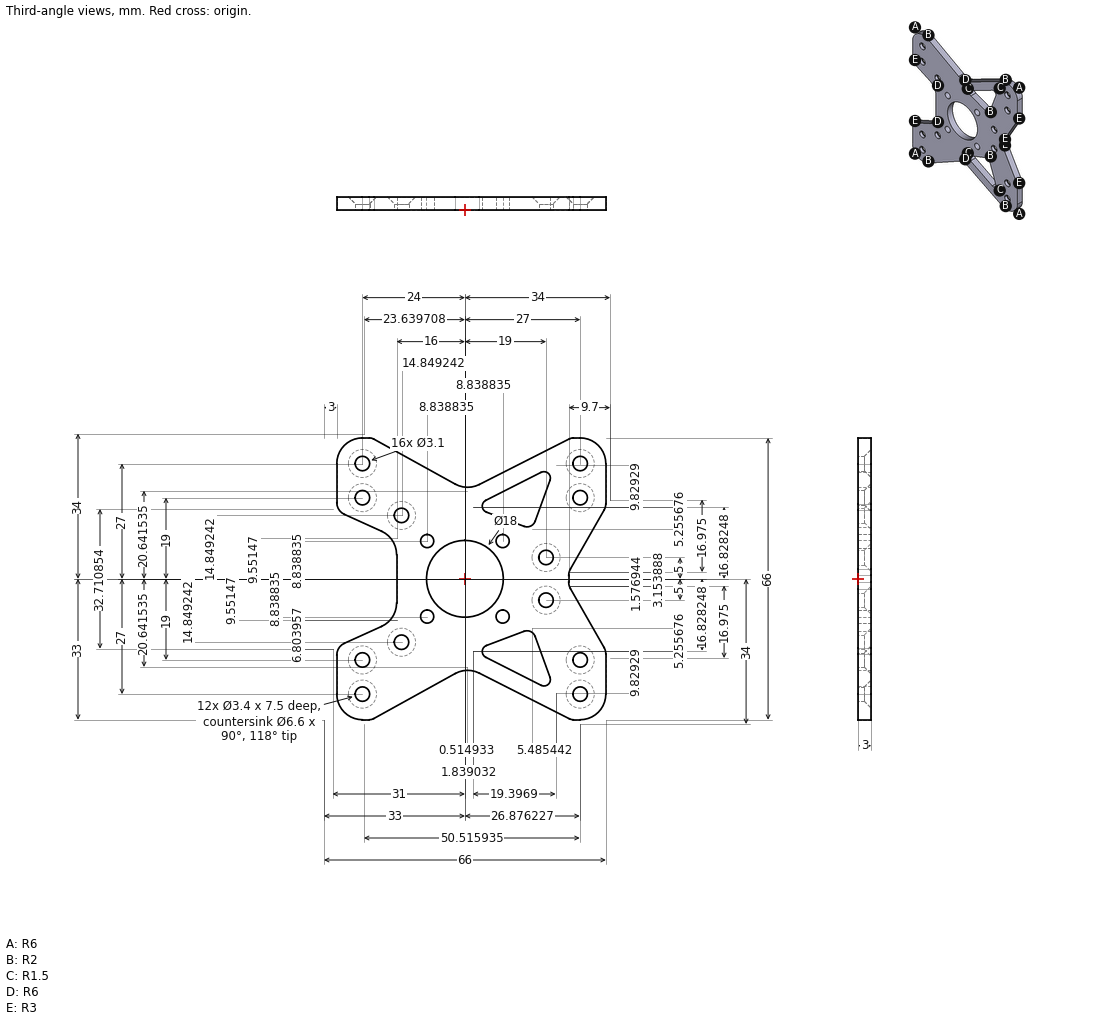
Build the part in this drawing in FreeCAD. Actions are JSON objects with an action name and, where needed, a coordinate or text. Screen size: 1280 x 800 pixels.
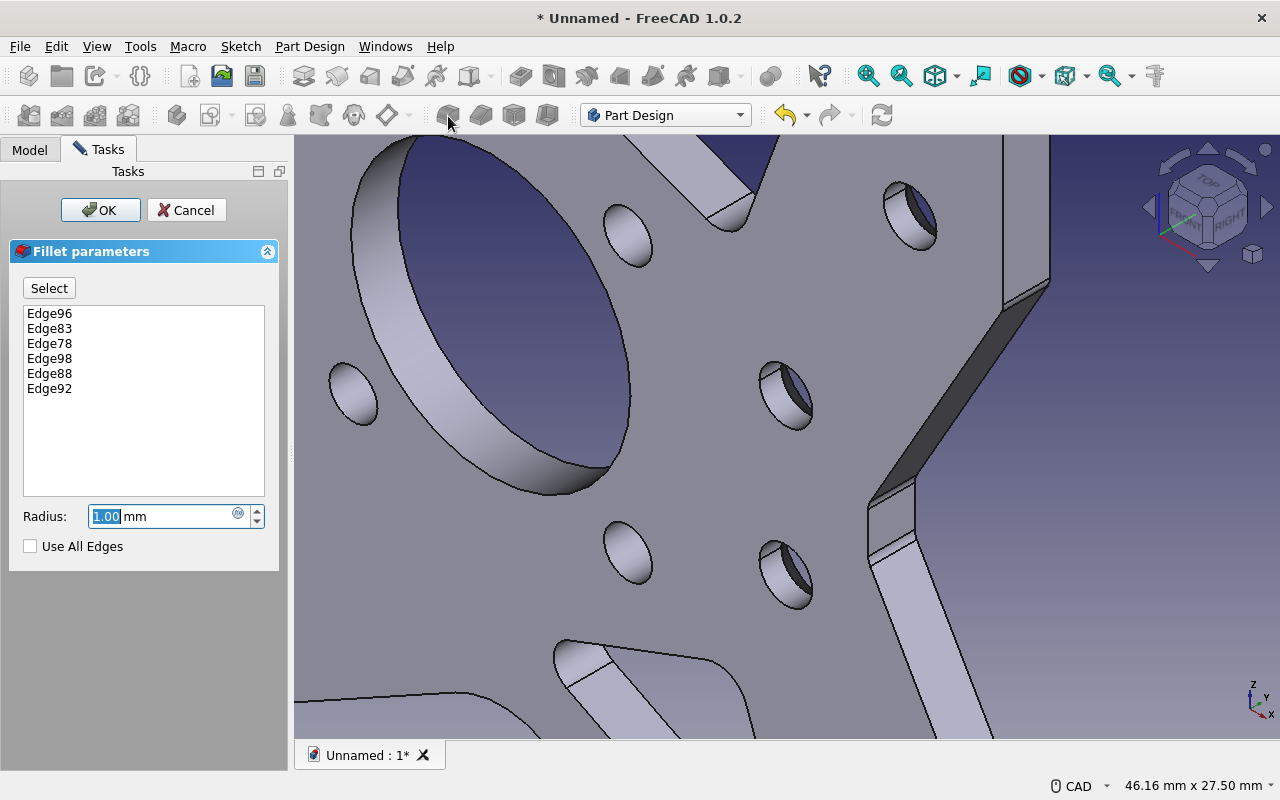
{"action": "type", "text": "3"}
{"action": "key", "text": "Tab"}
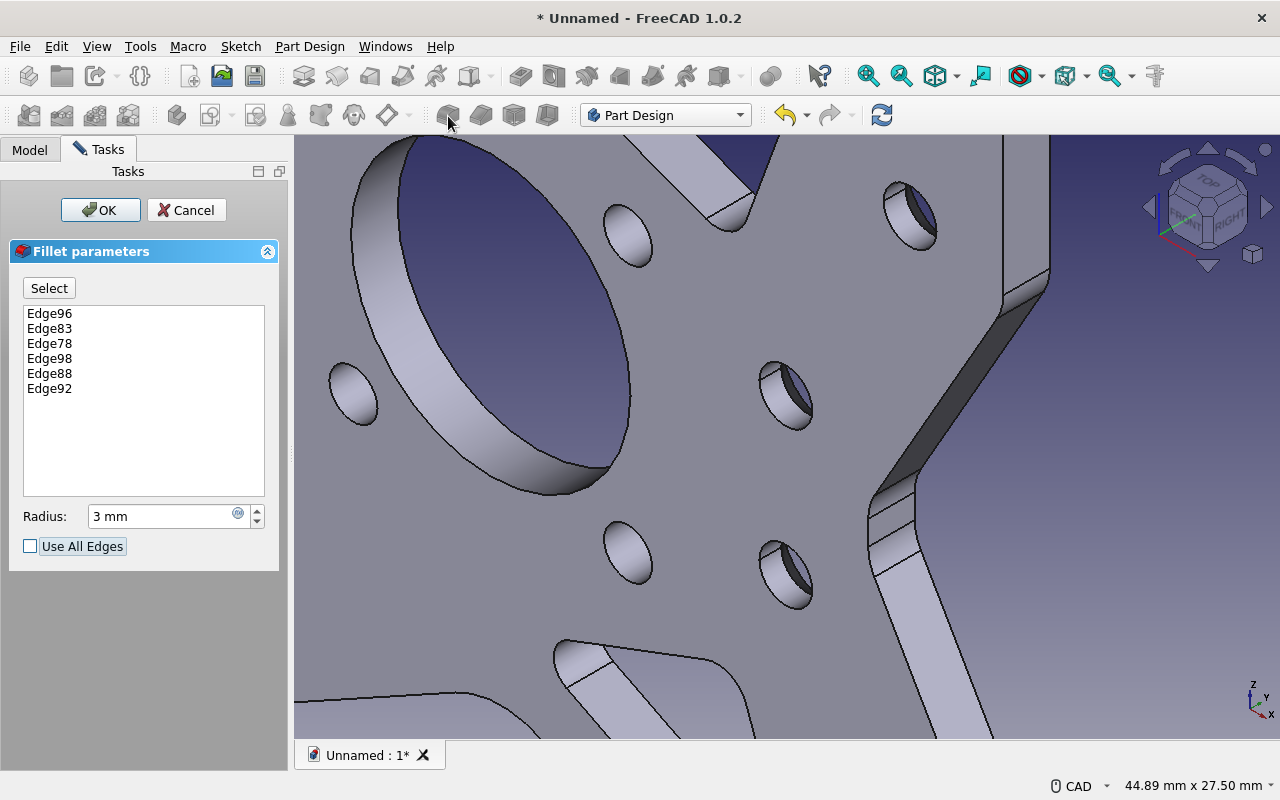
{"action": "left_click", "coordinate": [101, 210]}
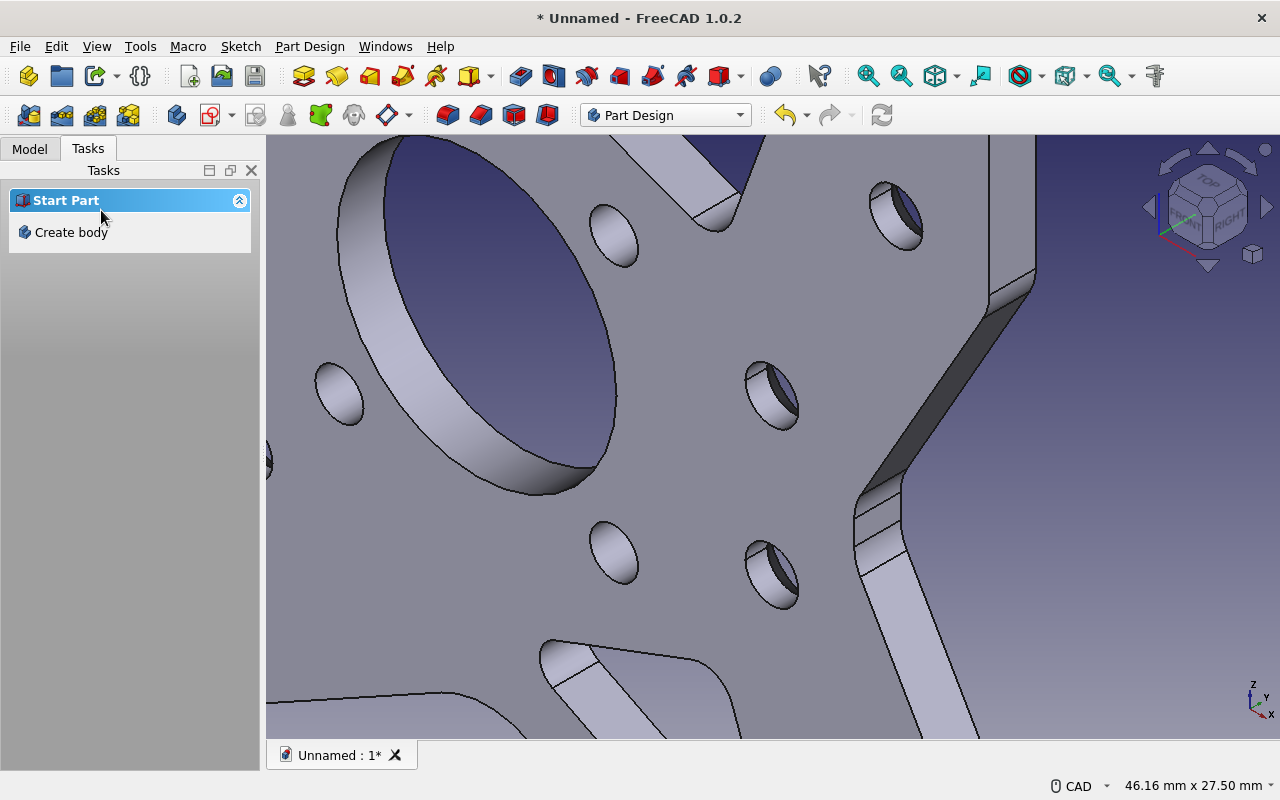
{"action": "left_click", "coordinate": [869, 76]}